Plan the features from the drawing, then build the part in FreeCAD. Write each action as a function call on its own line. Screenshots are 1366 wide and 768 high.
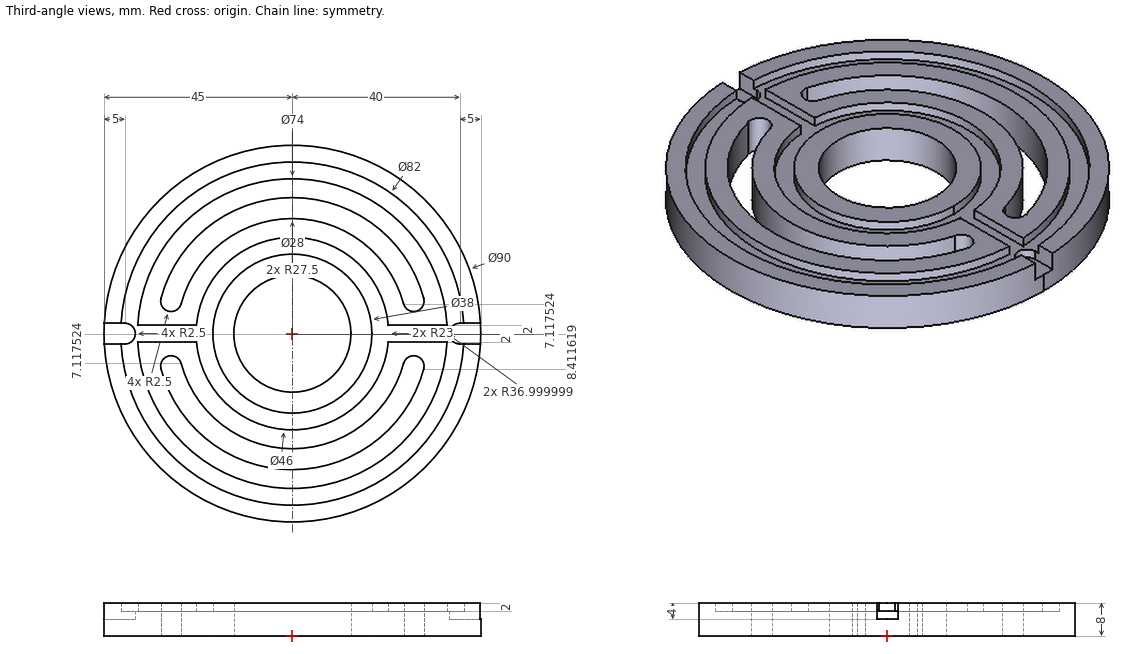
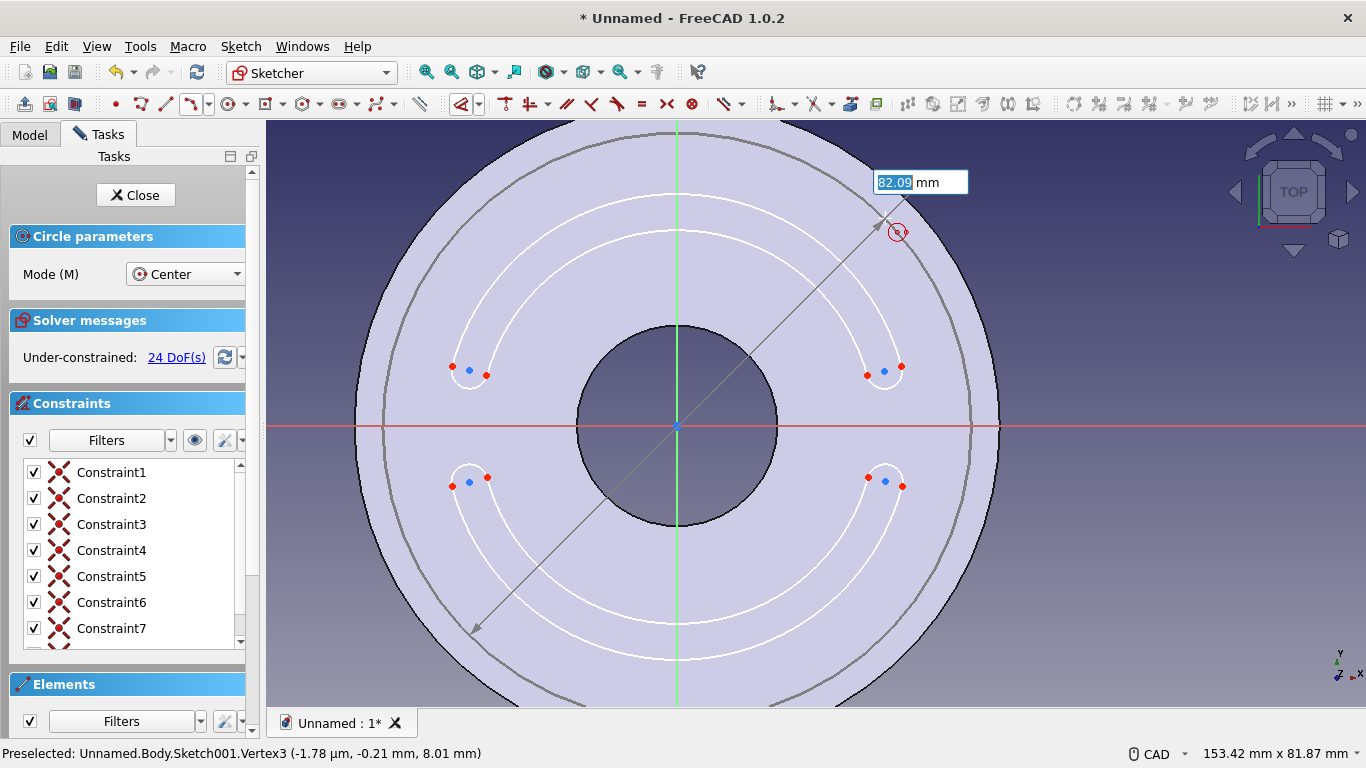
text(82)
key(Return)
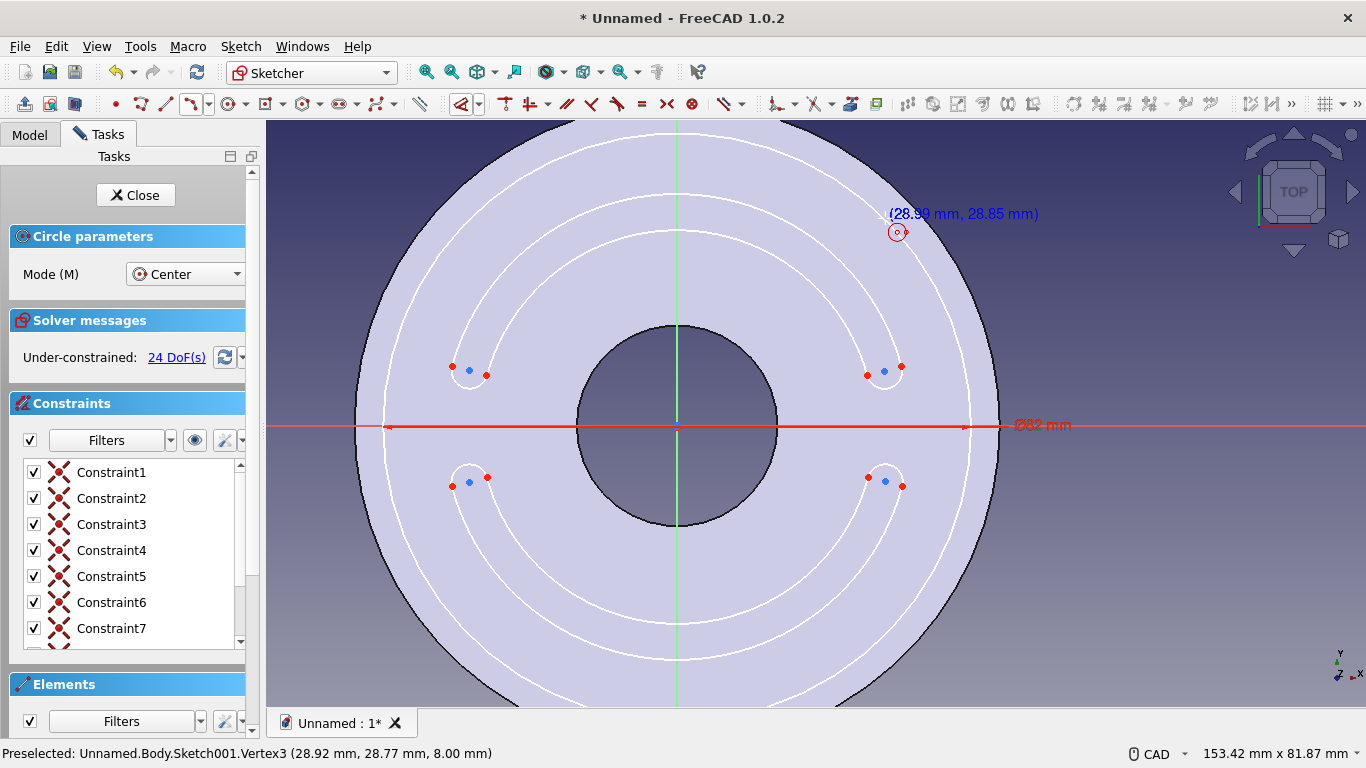
click(678, 426)
move(794, 309)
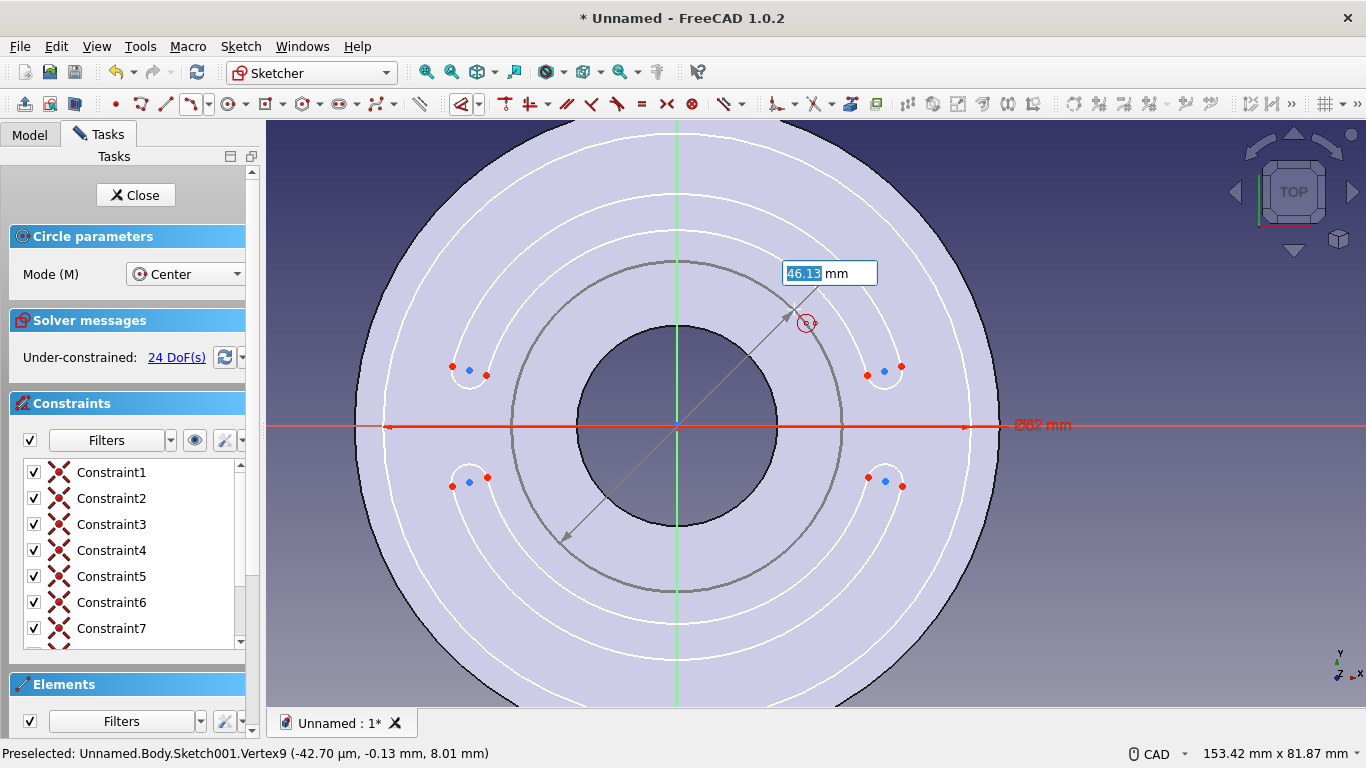
text(46)
key(Return)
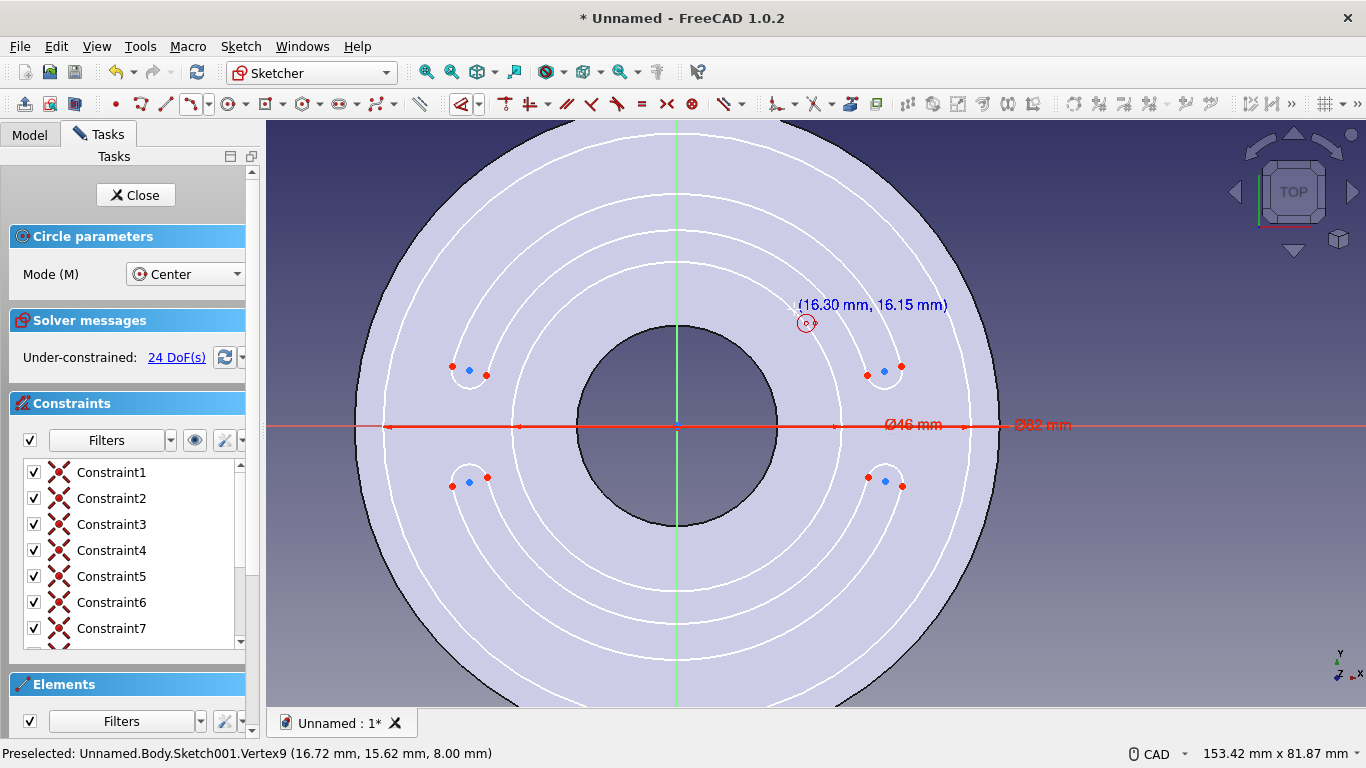
click(678, 426)
move(865, 238)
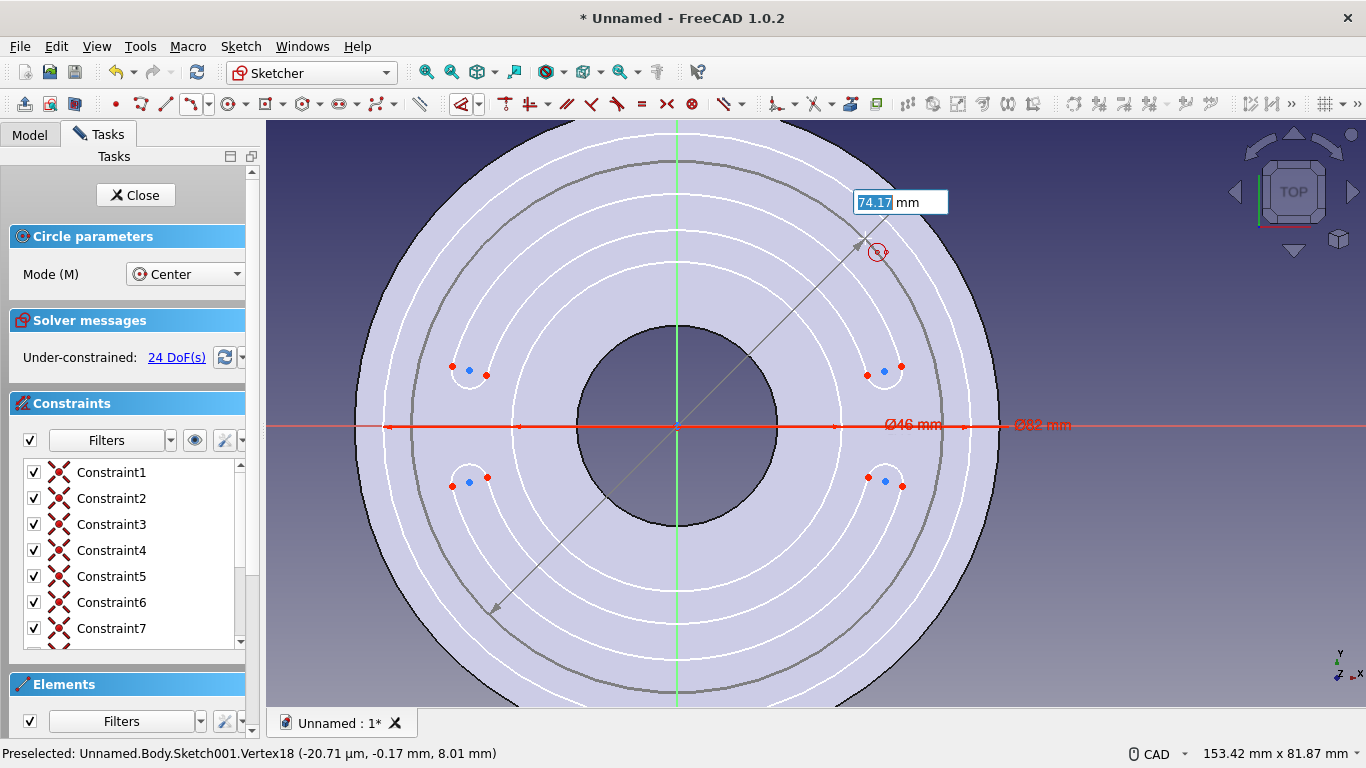
text(74)
key(Return)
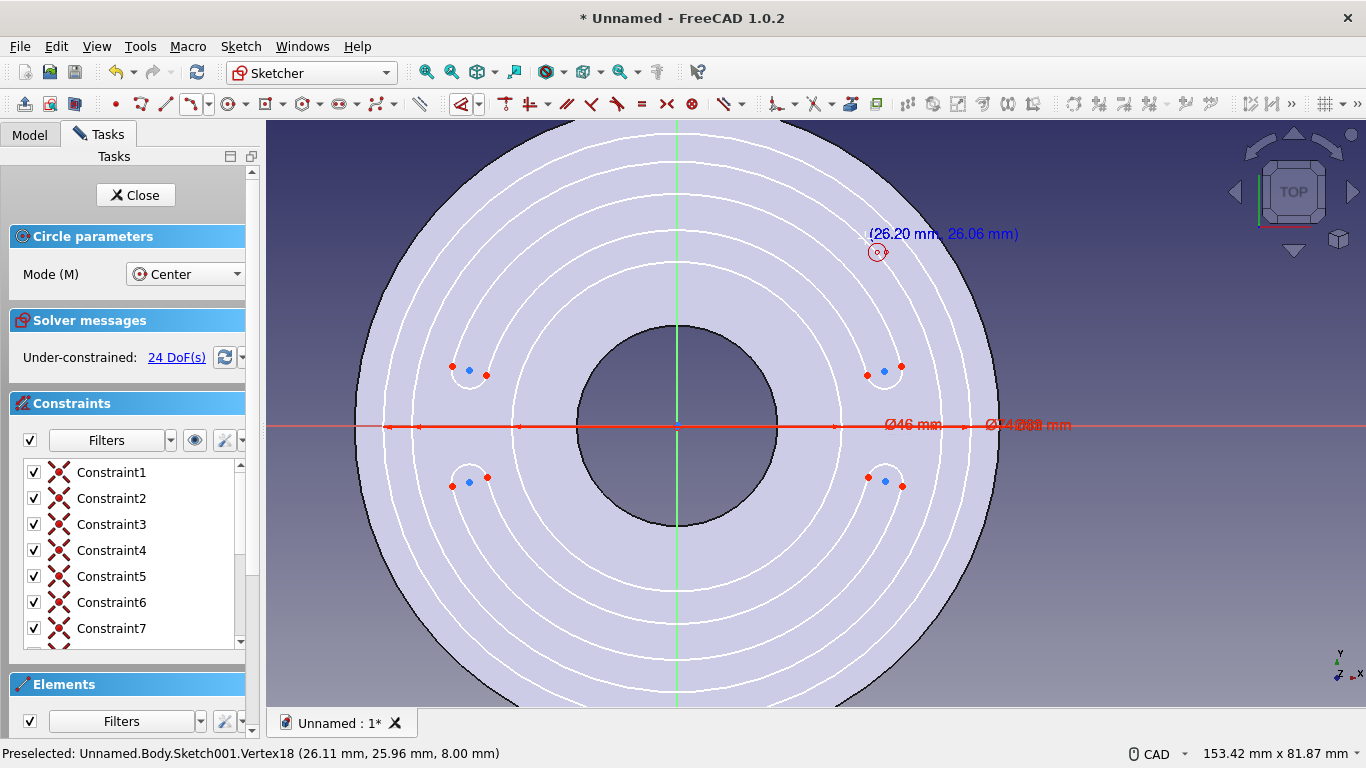
click(678, 426)
move(773, 329)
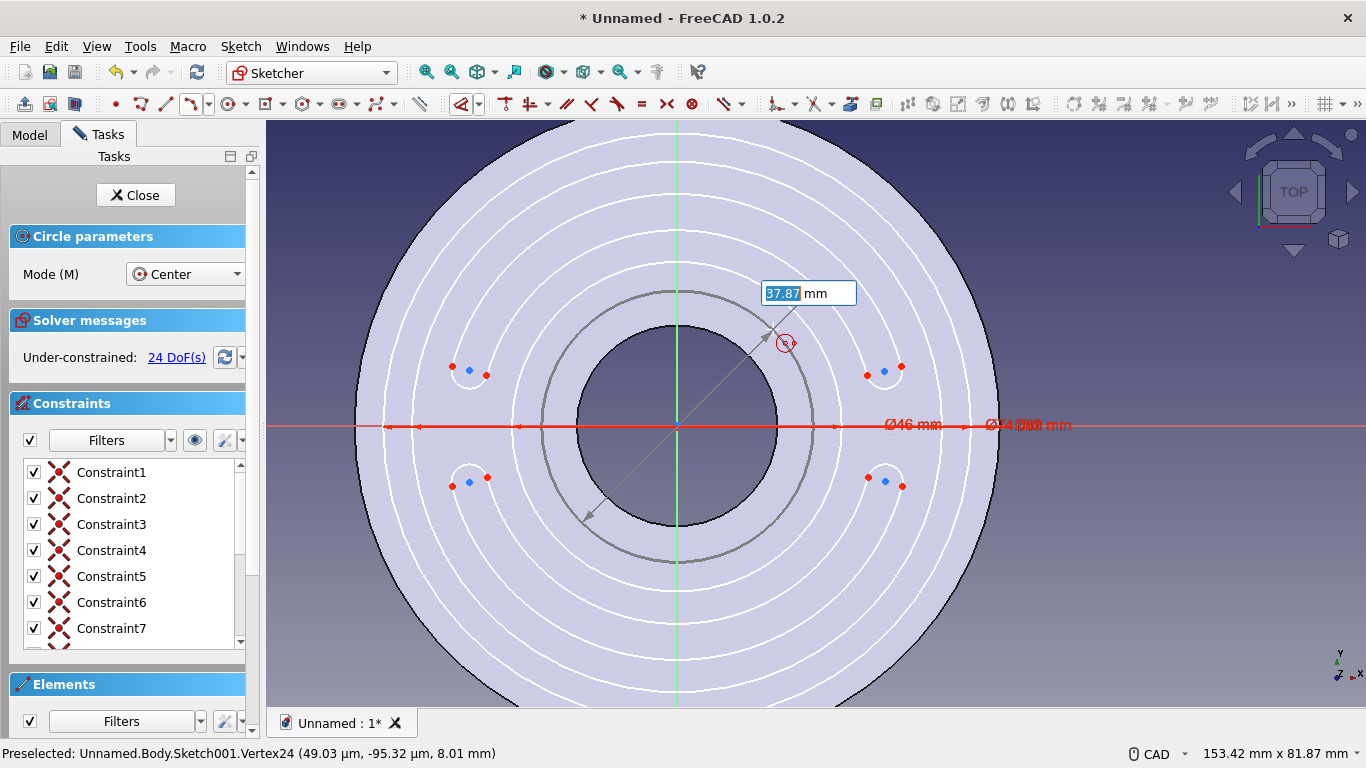
text(38)
key(Return)
key(Escape)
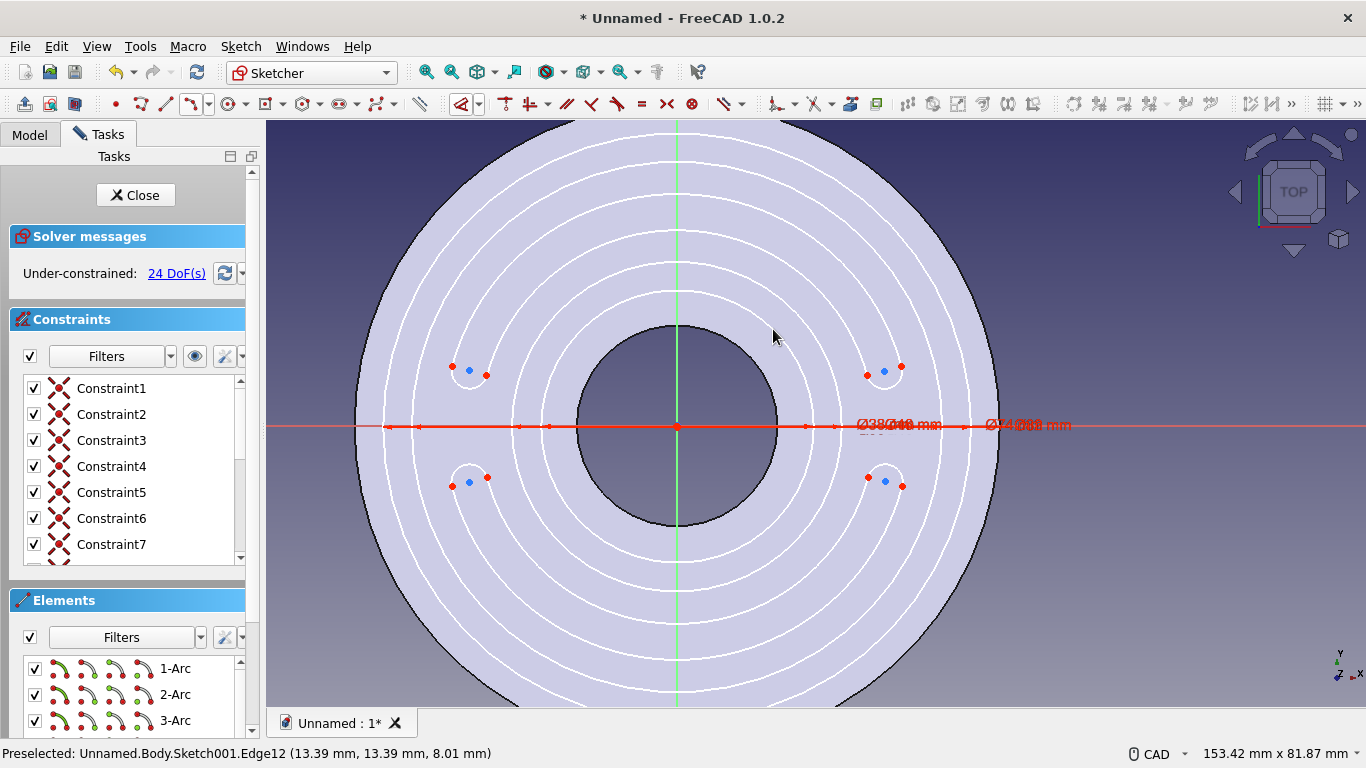
click(775, 257)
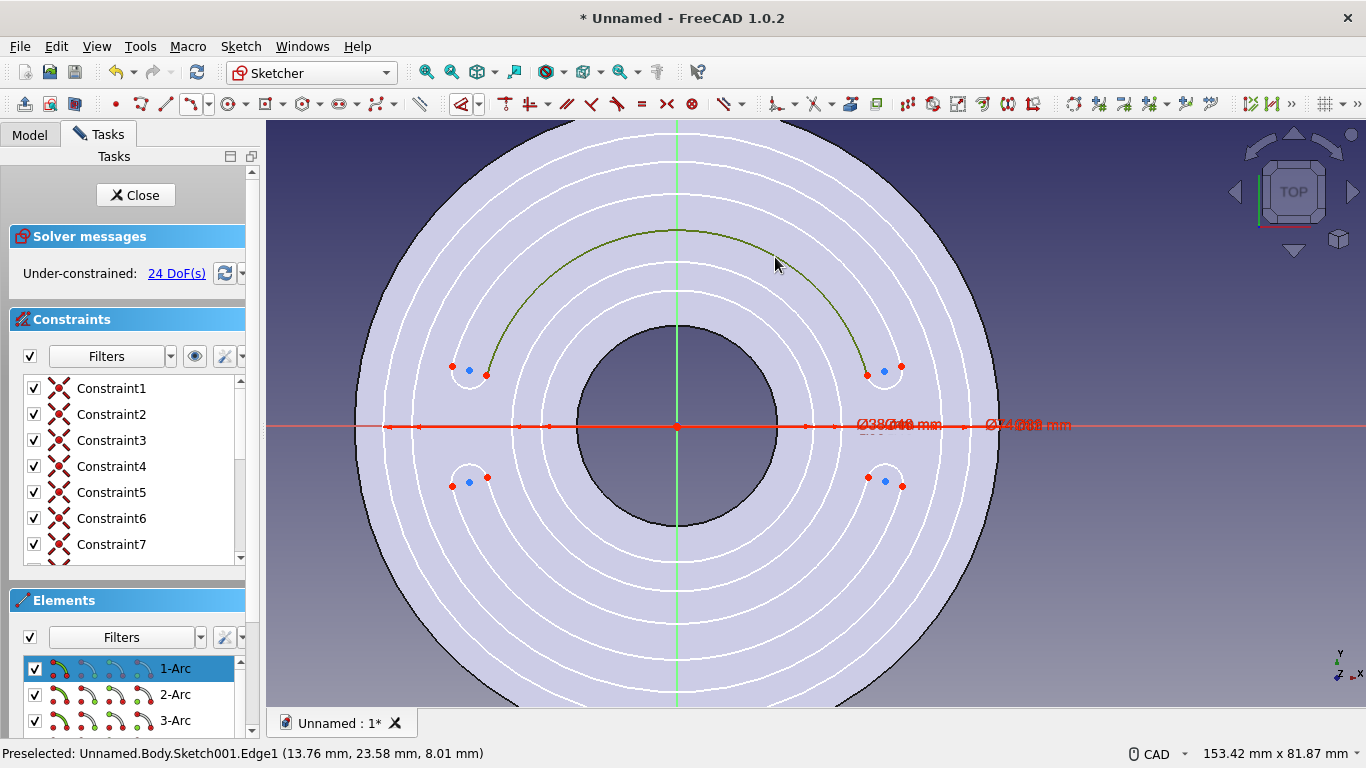
click(878, 388)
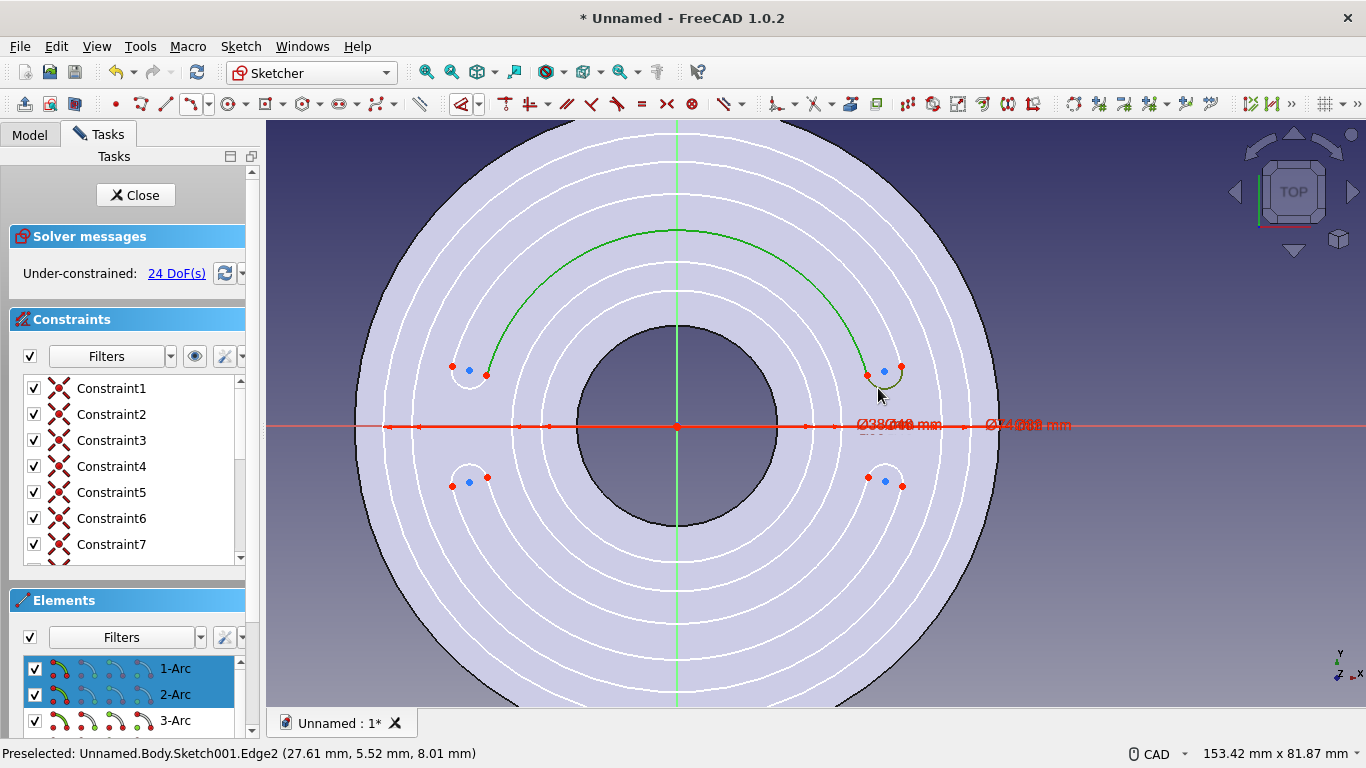
key(t)